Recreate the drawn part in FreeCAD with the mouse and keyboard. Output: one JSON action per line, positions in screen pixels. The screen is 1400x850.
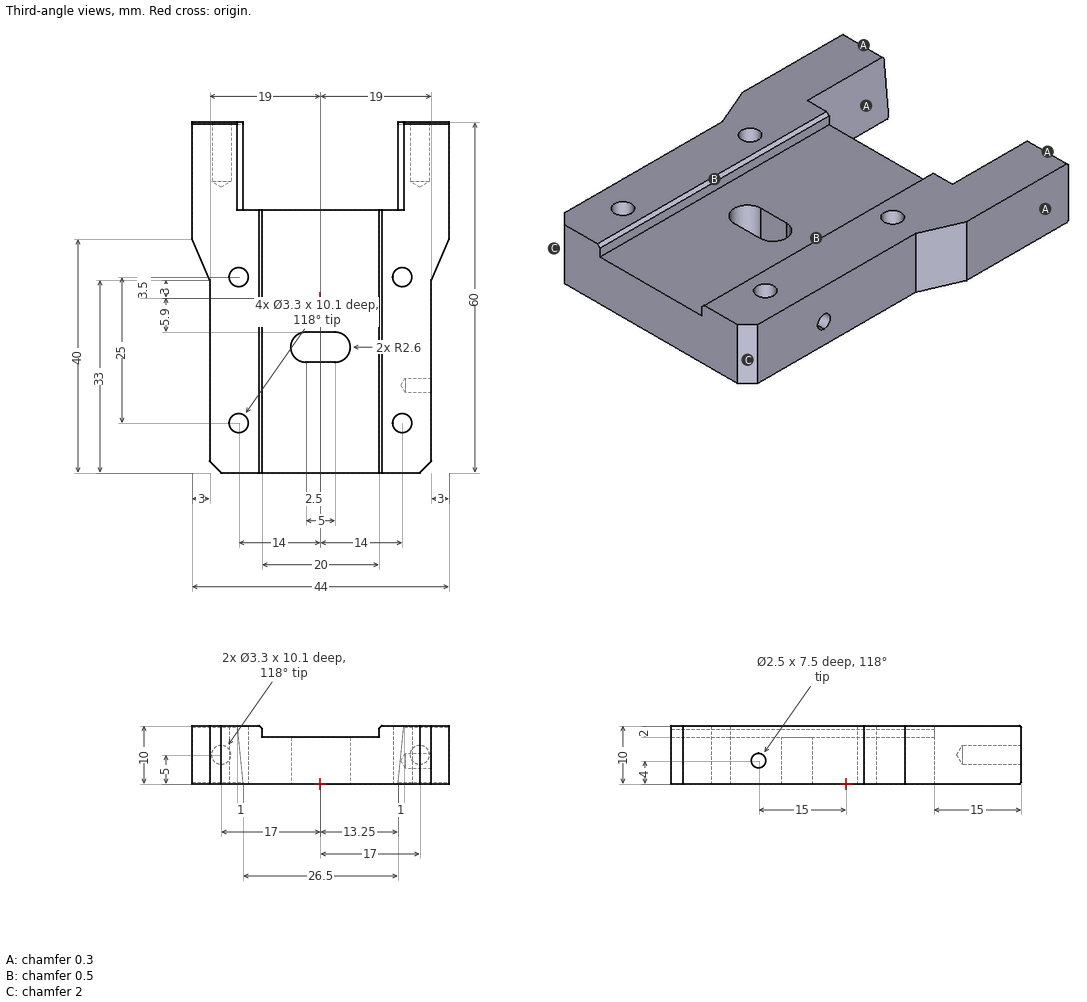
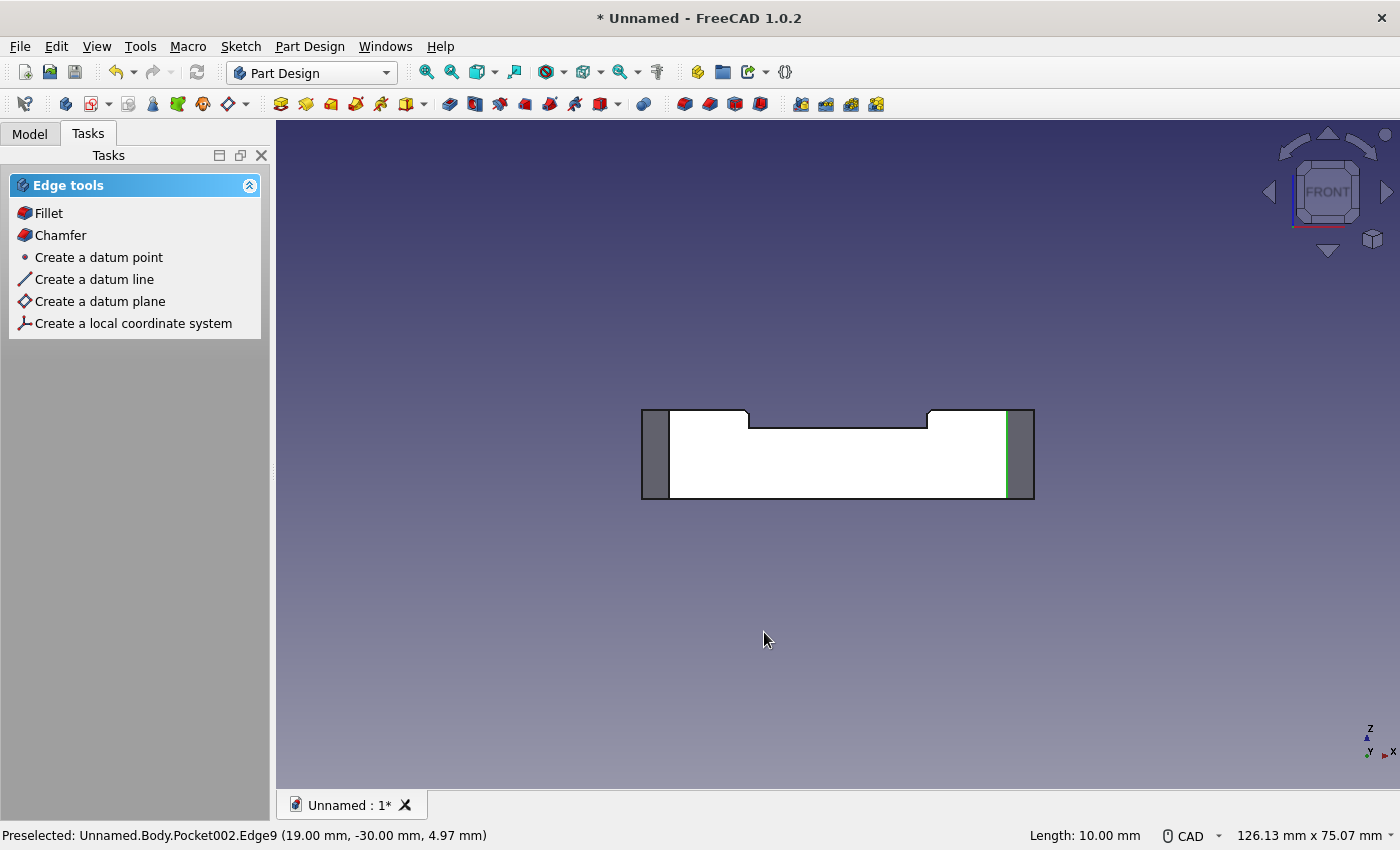
{"action": "left_click", "coordinate": [427, 72]}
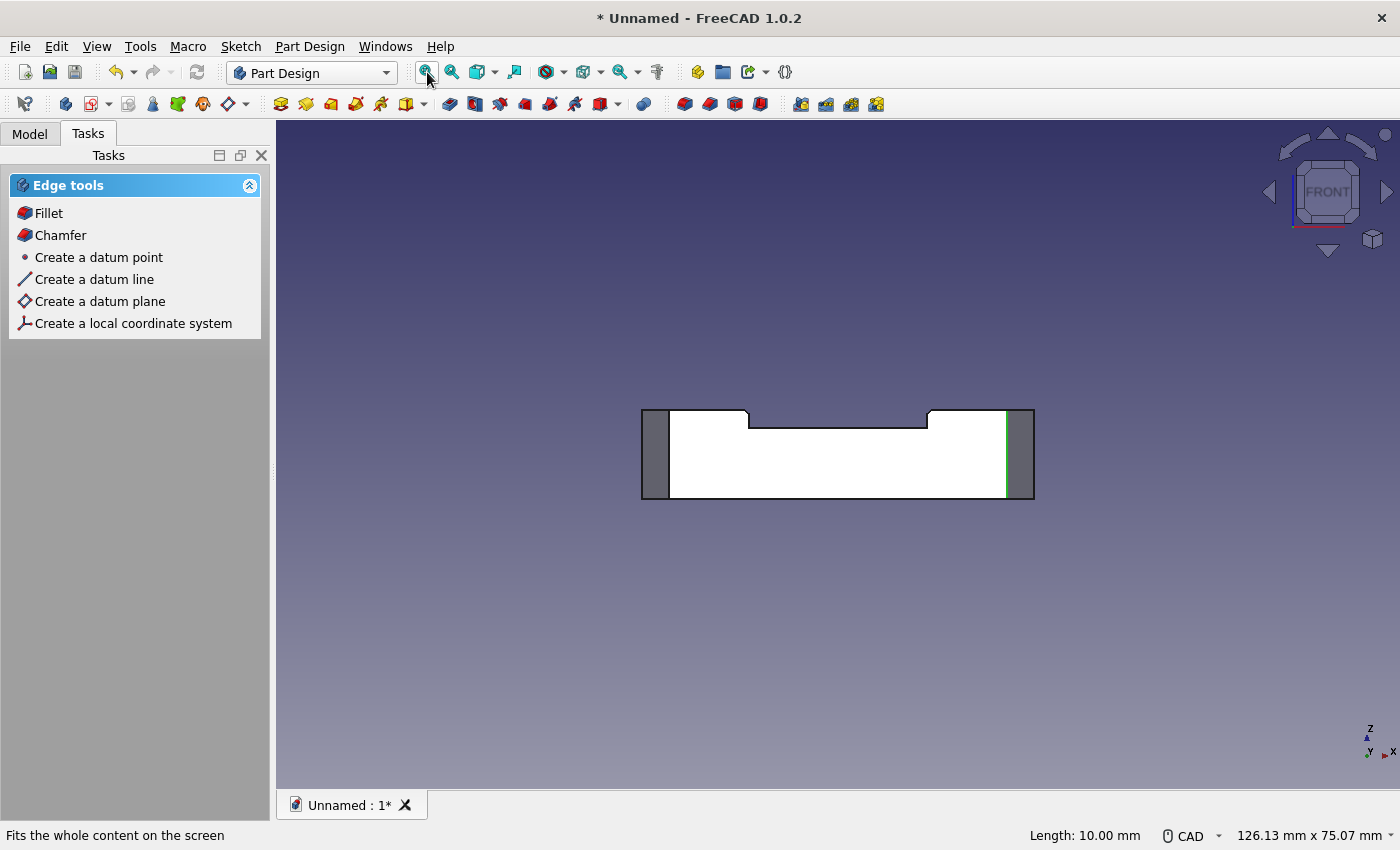
{"action": "left_click", "coordinate": [669, 454], "text": "ctrl"}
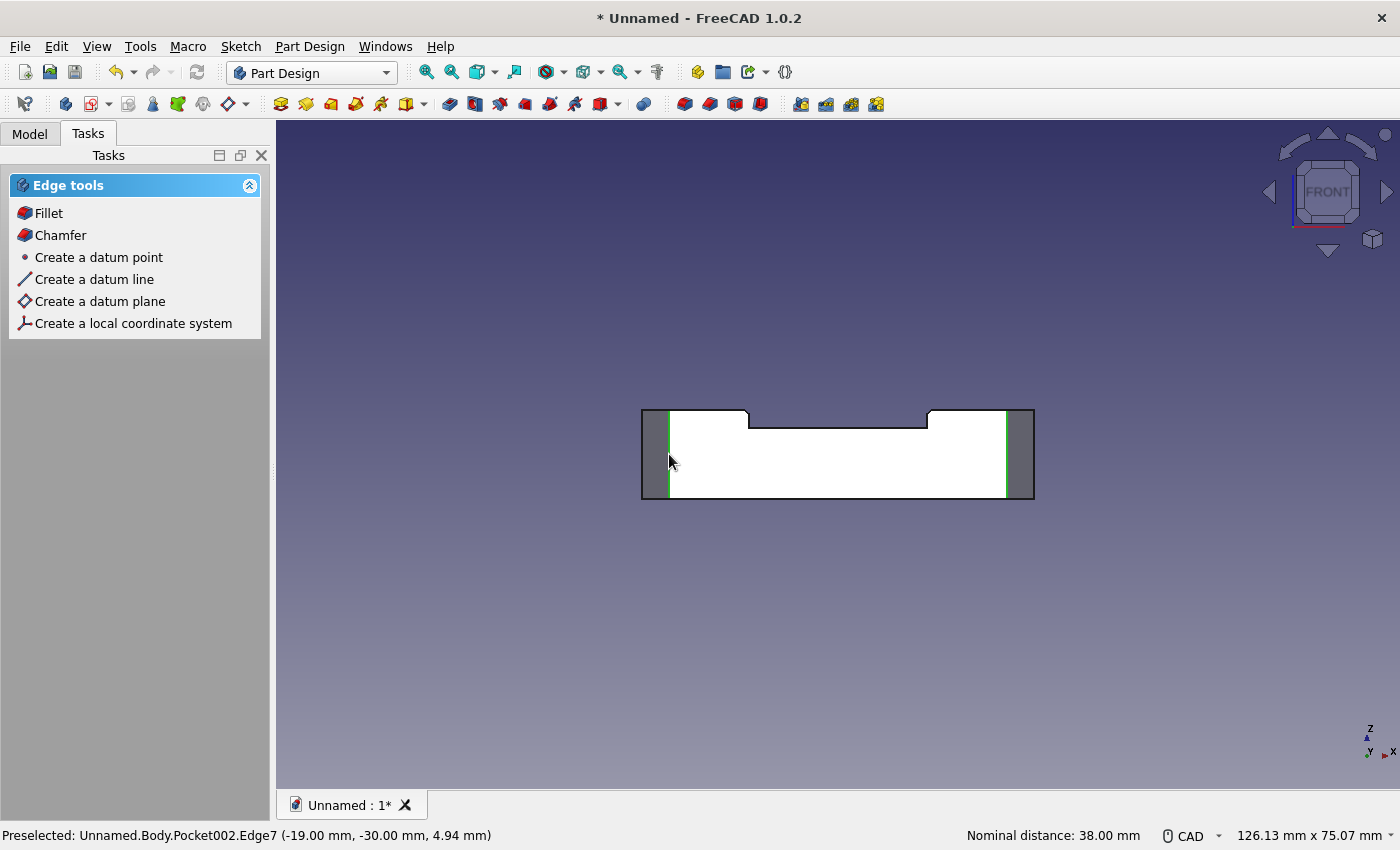
{"action": "left_click", "coordinate": [710, 104]}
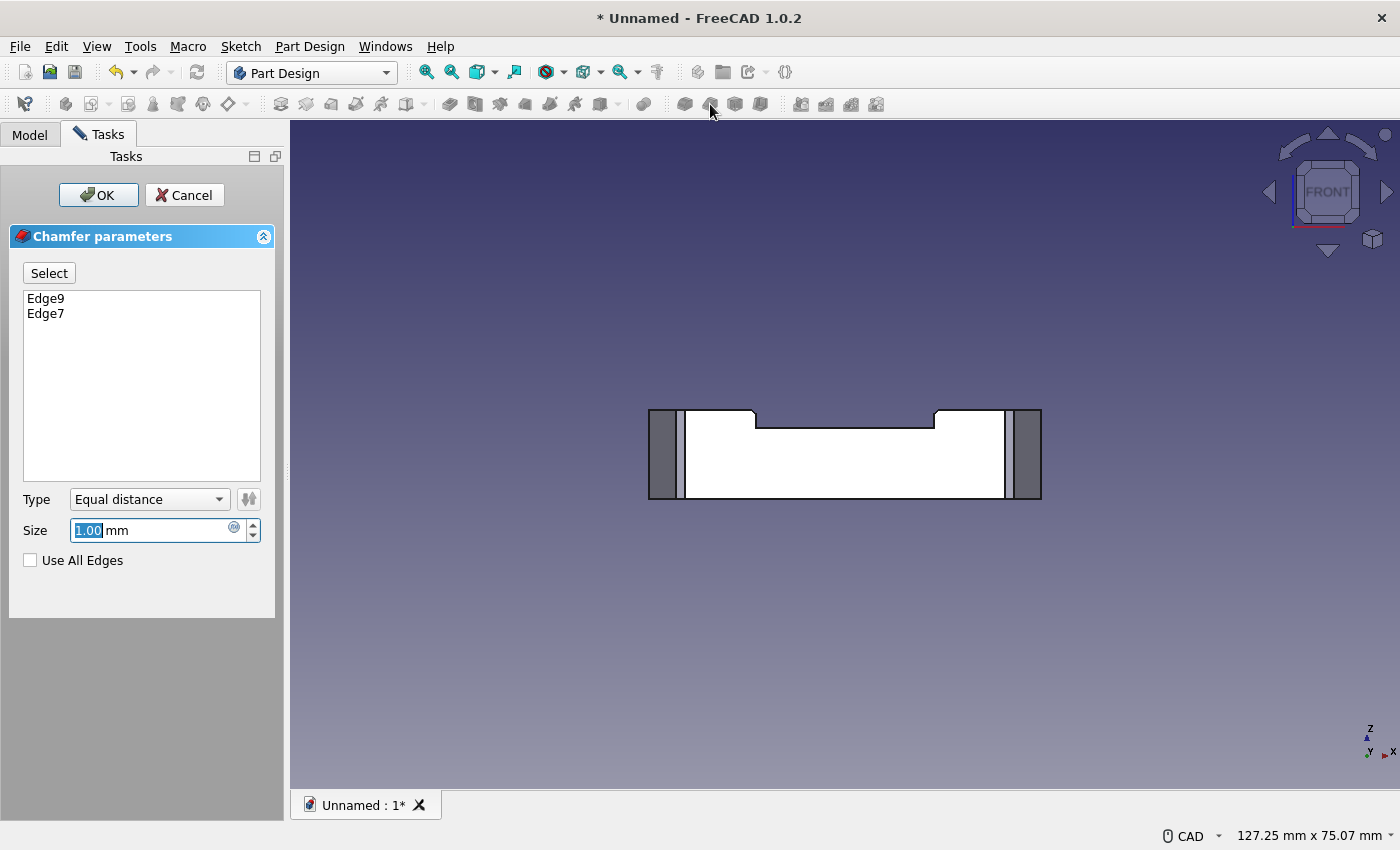
{"action": "type", "text": "2"}
{"action": "key", "text": "Tab"}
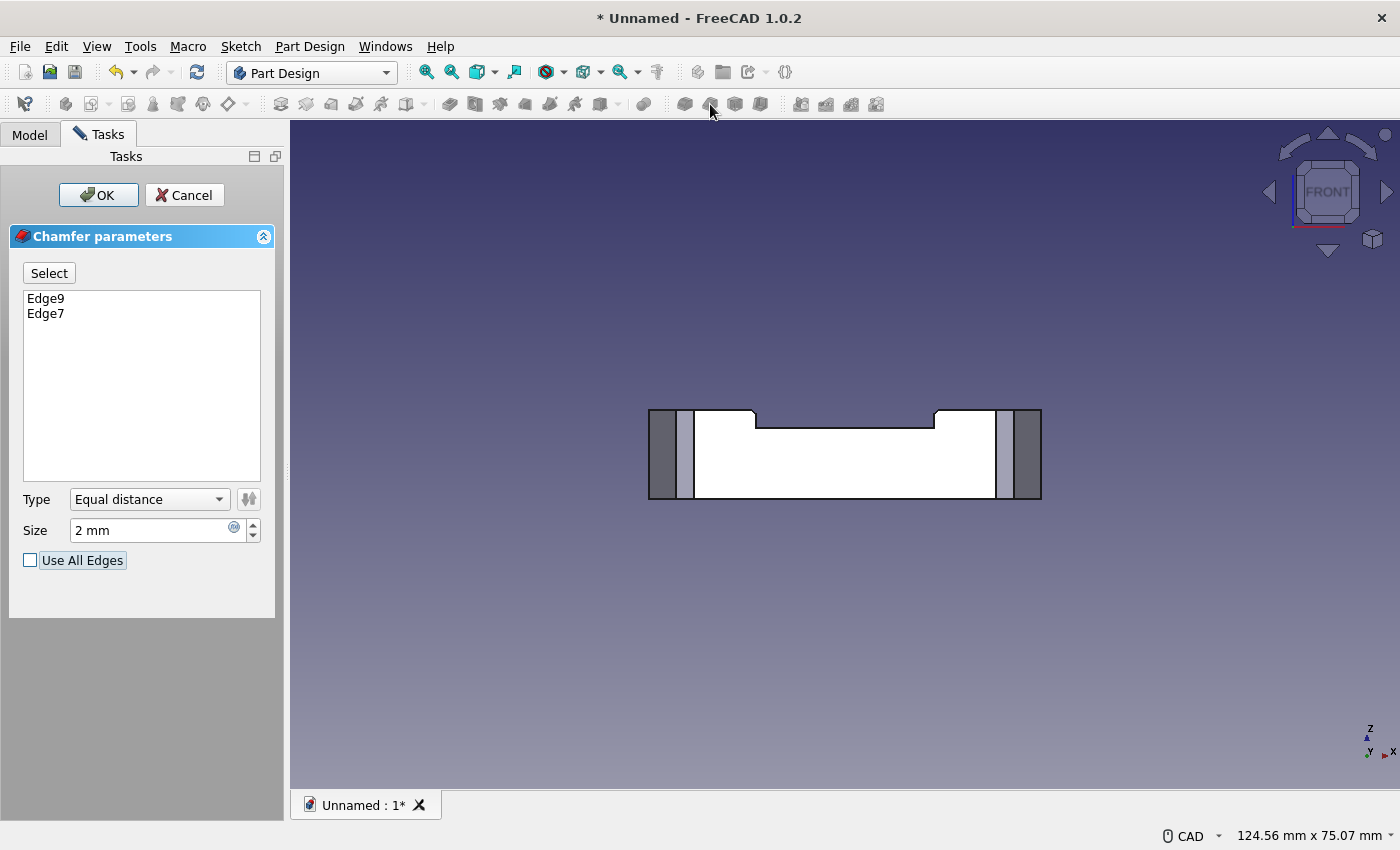
{"action": "left_click", "coordinate": [99, 195]}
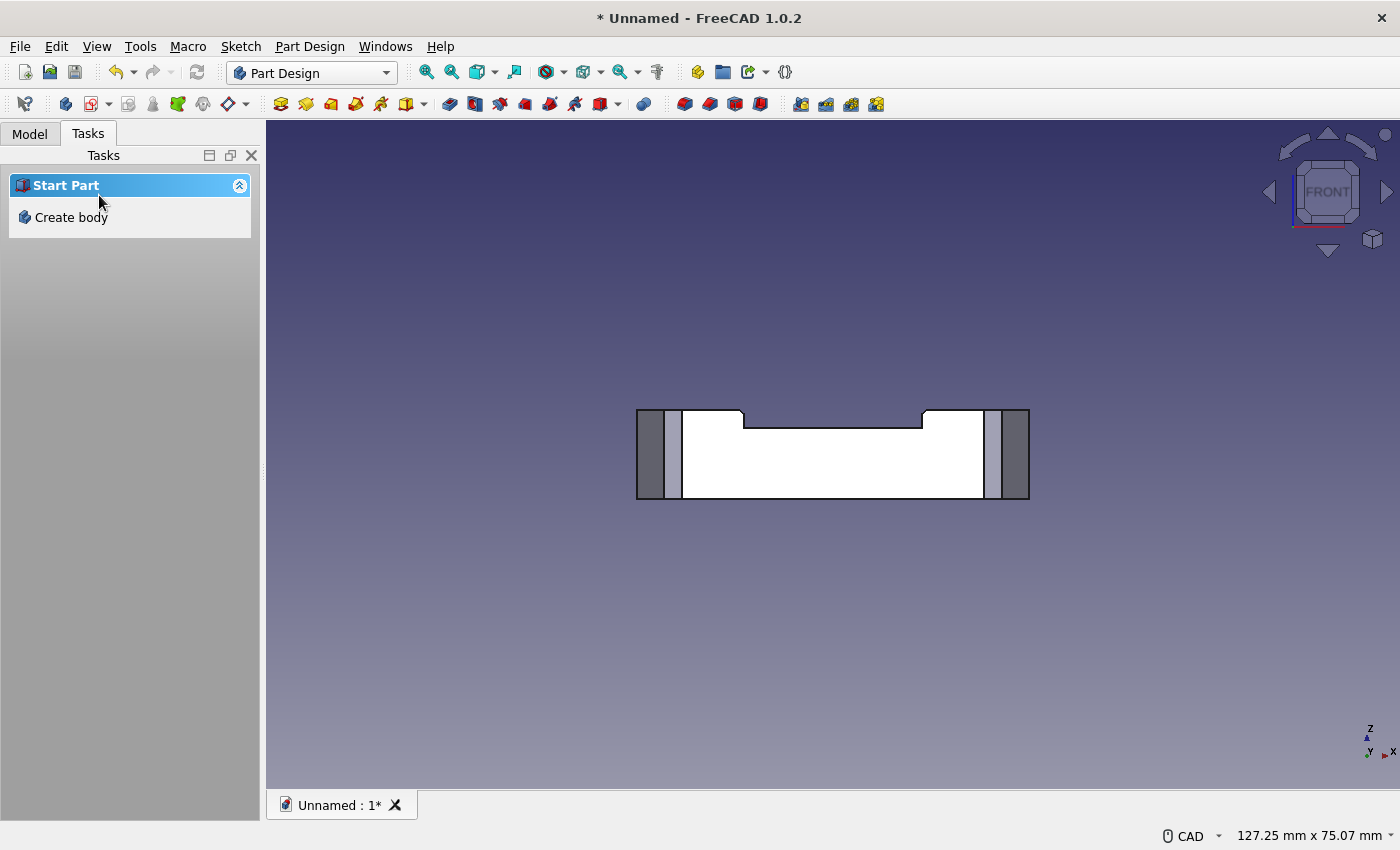
{"action": "left_click", "coordinate": [427, 72]}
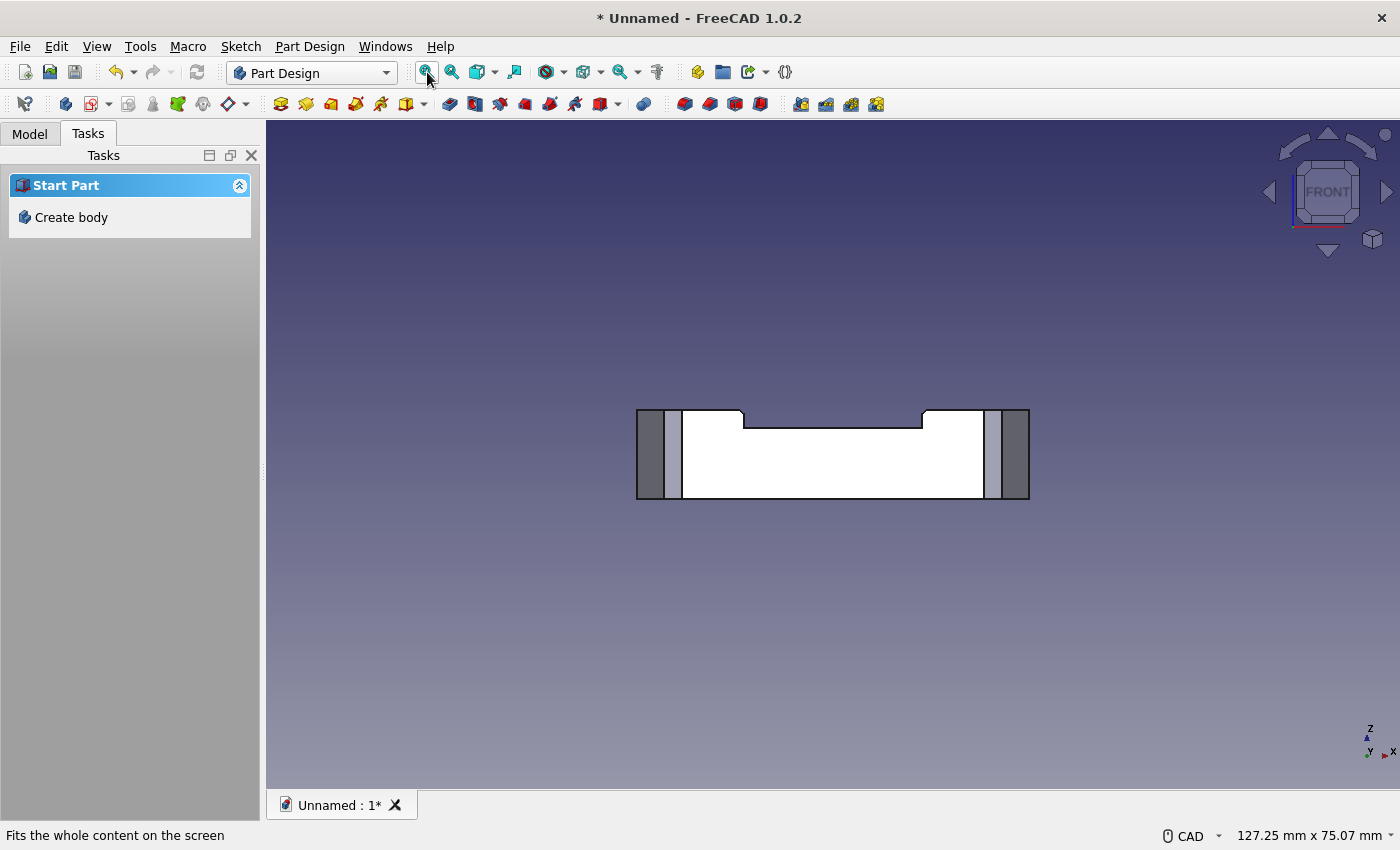
{"action": "key", "text": "5"}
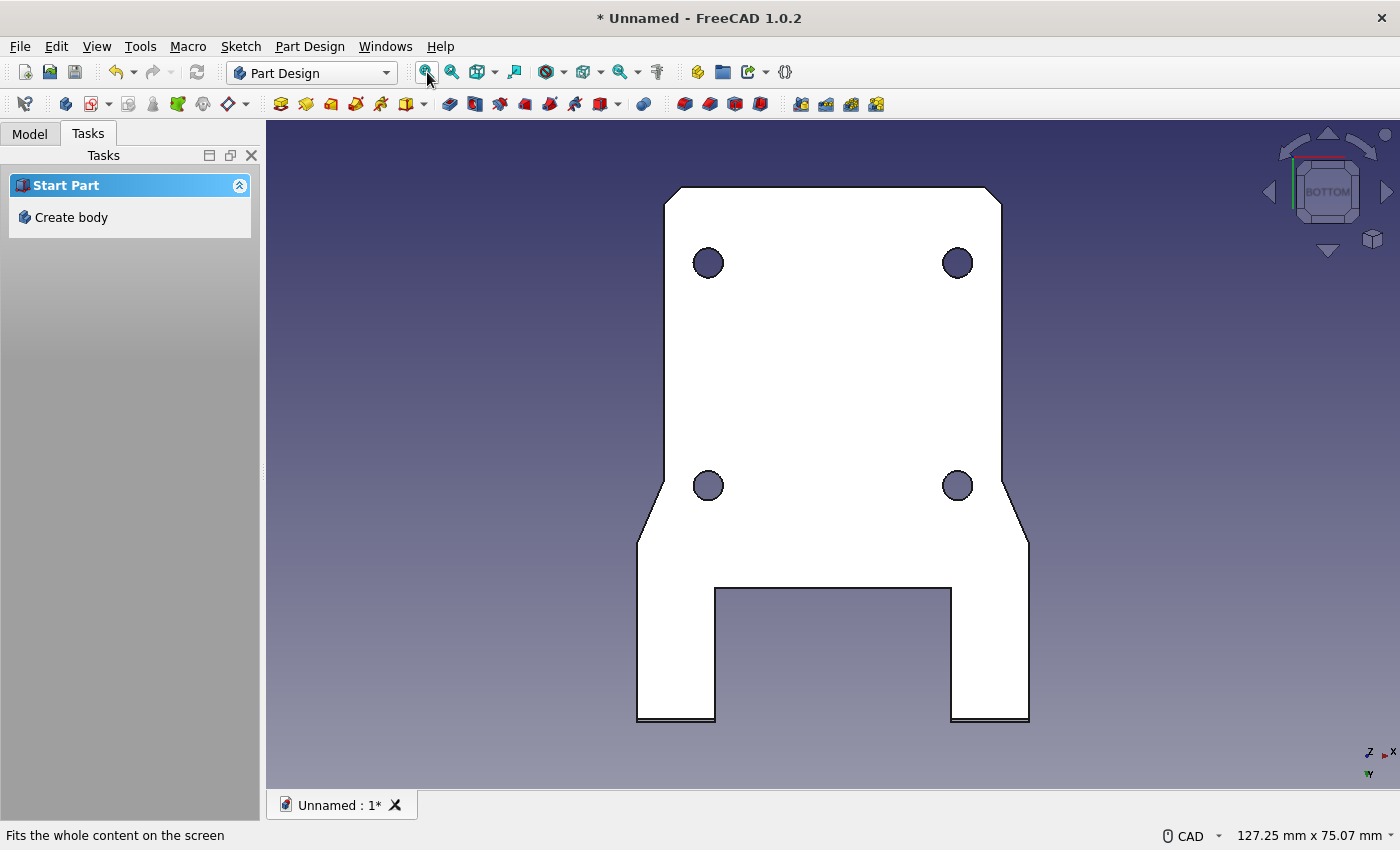
{"action": "left_click", "coordinate": [833, 376]}